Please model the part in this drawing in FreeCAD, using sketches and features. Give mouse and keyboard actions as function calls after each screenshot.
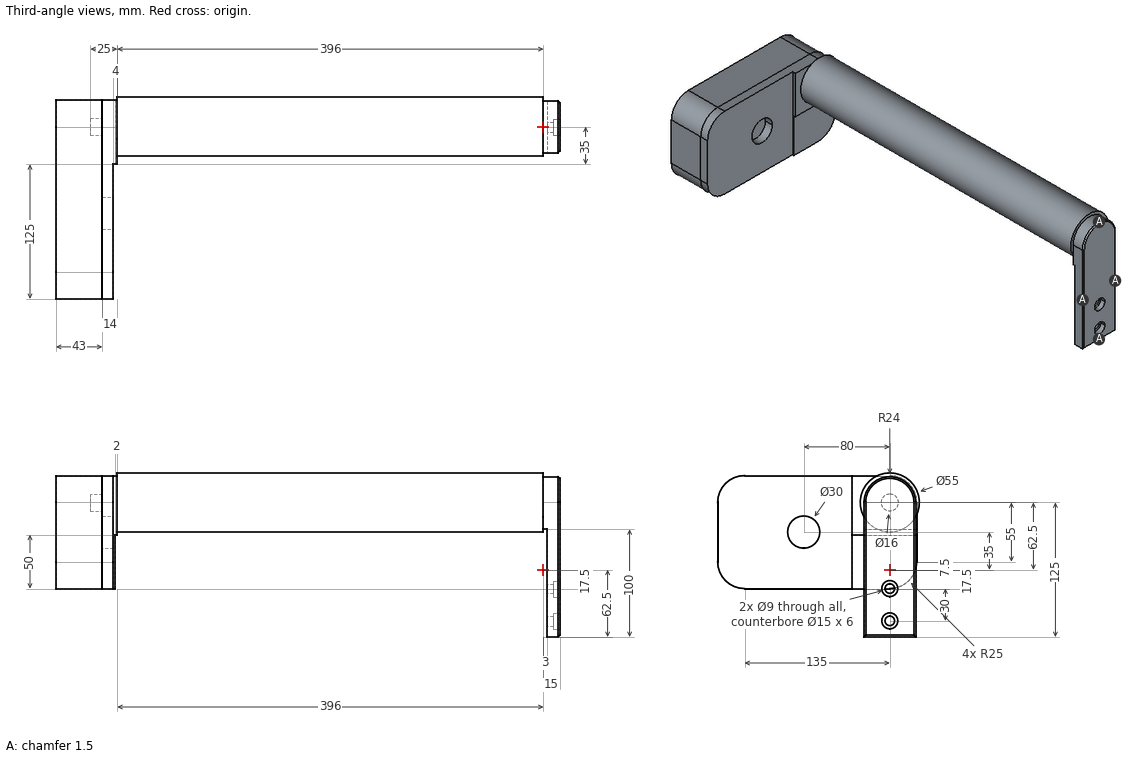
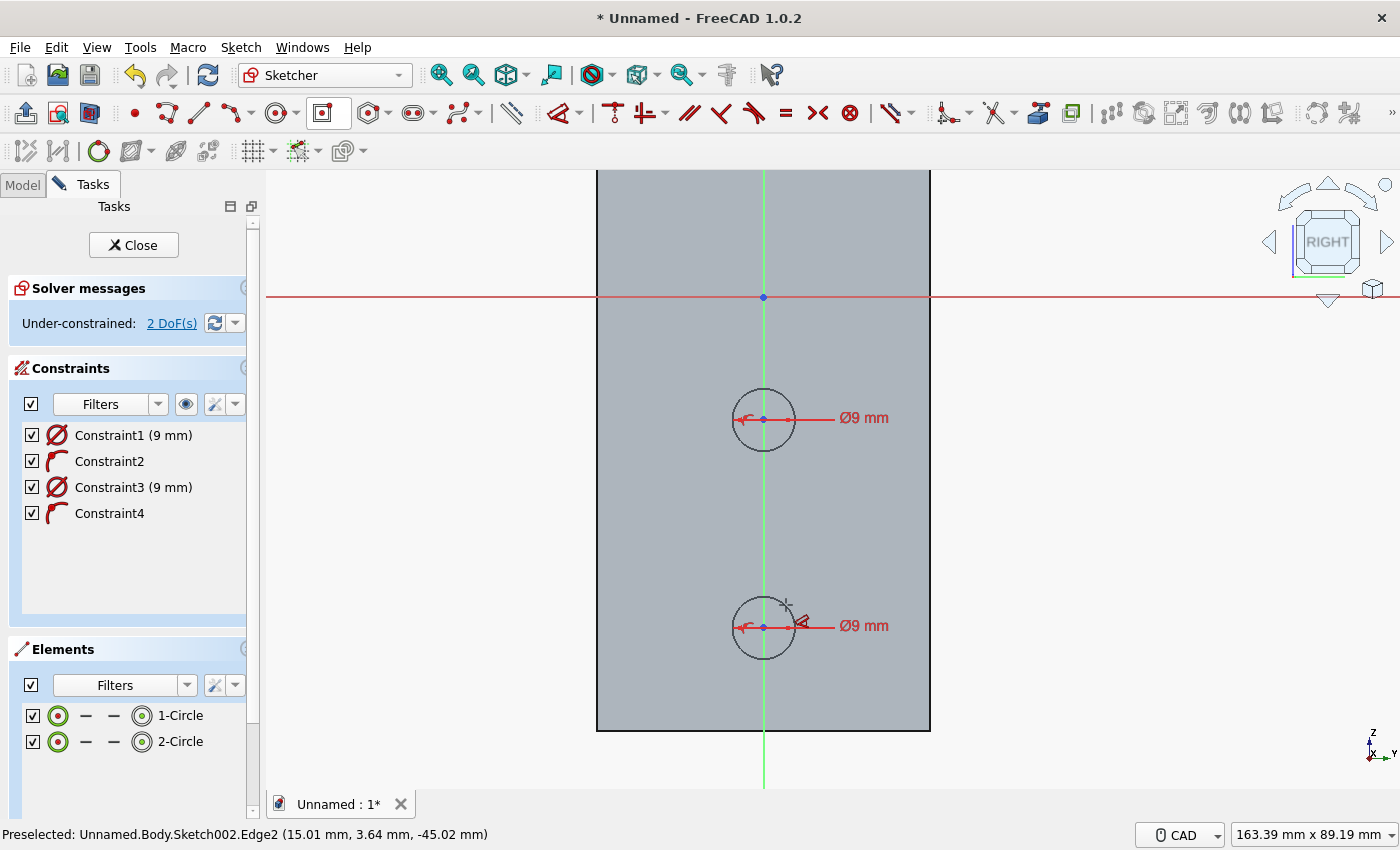
click(764, 420)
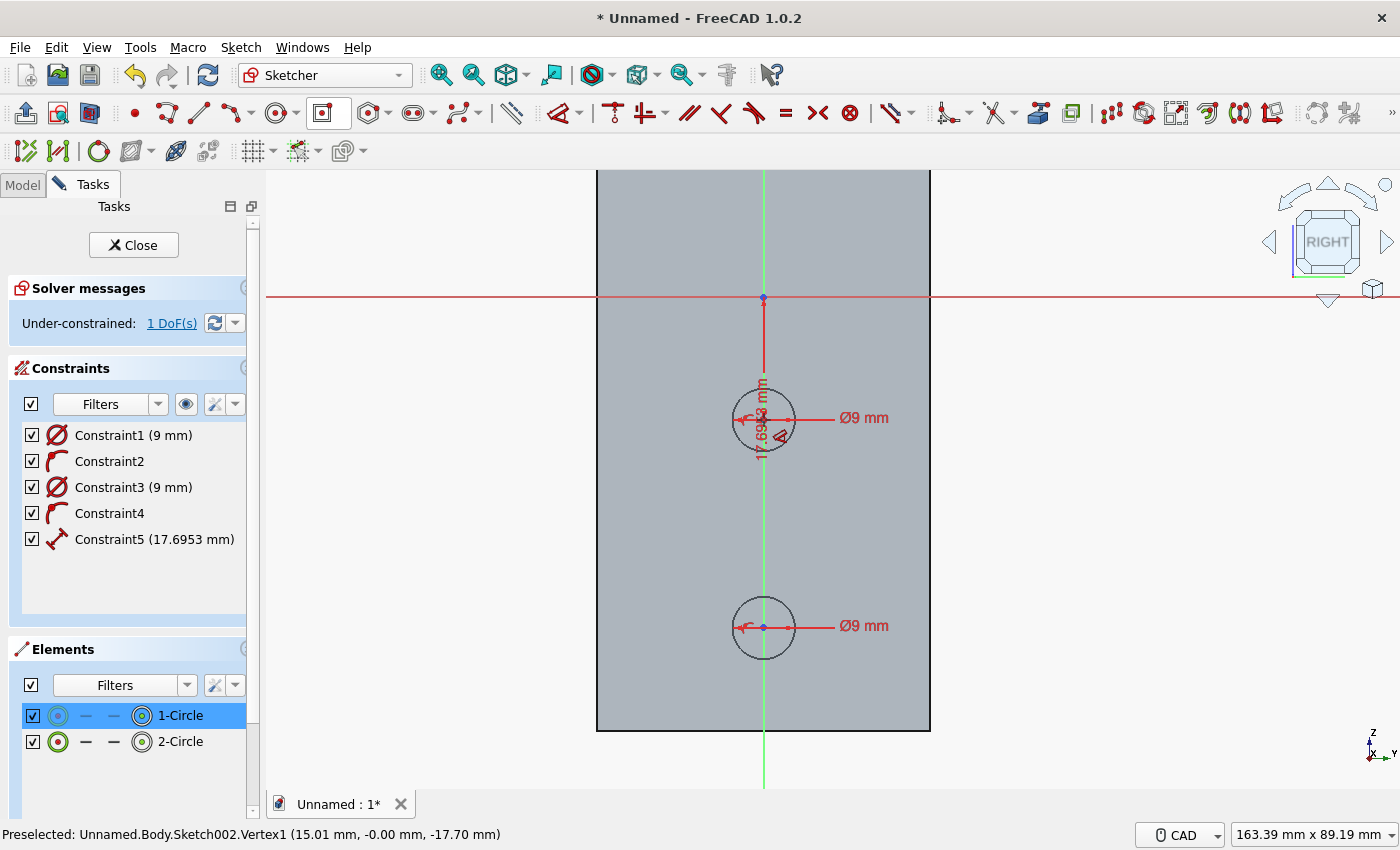
click(764, 628)
click(798, 524)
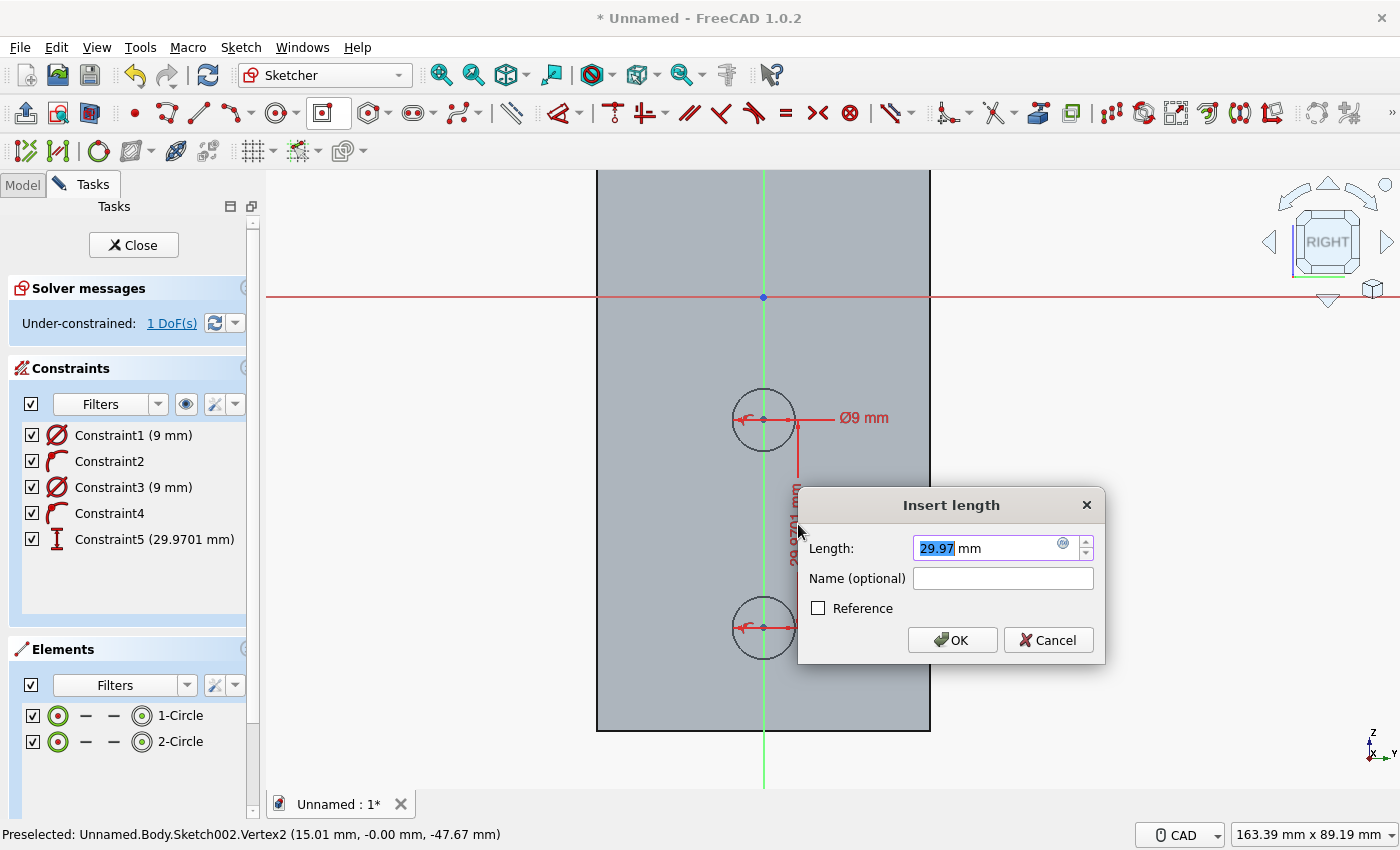
text(30)
key(Return)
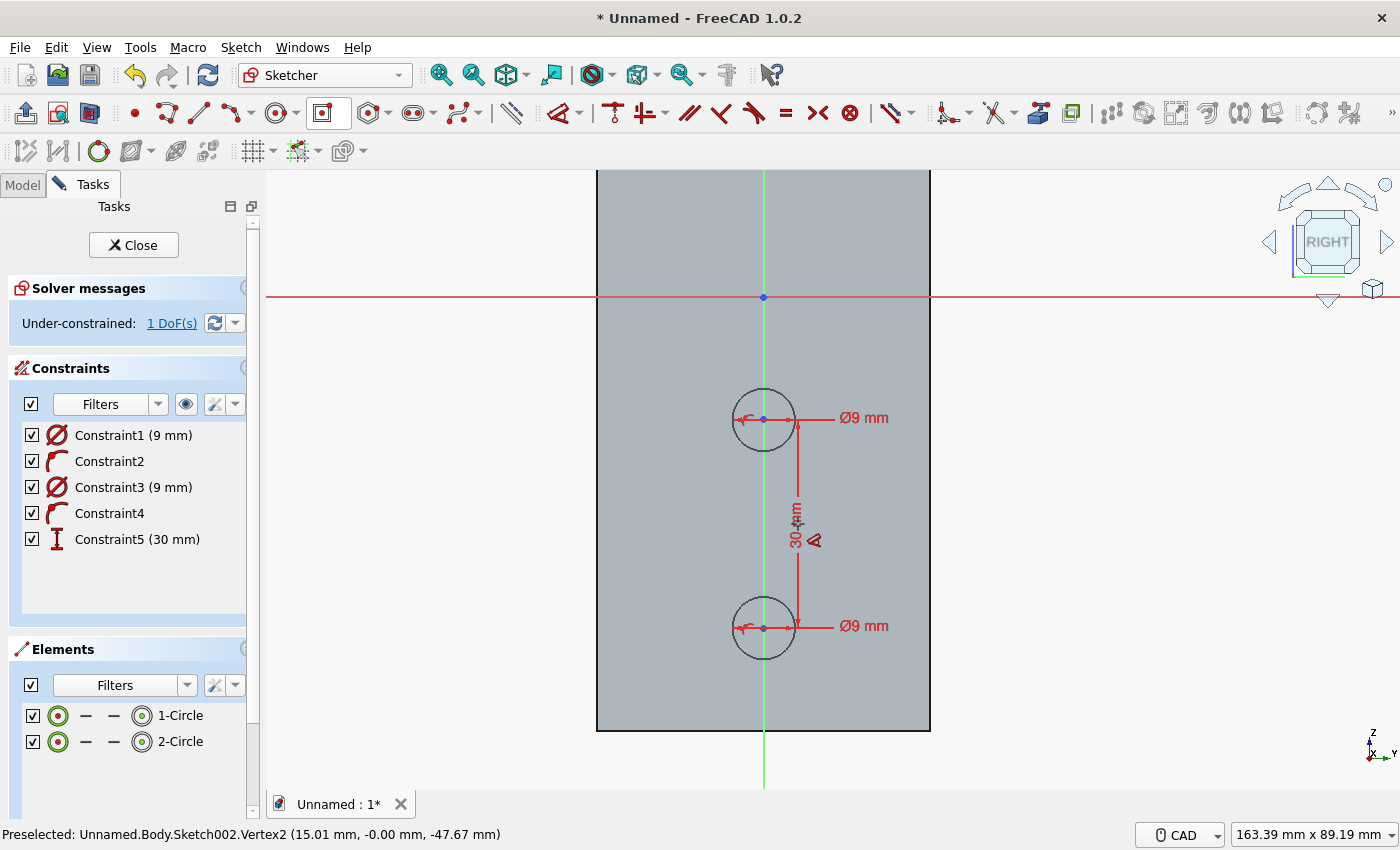
click(764, 420)
click(798, 359)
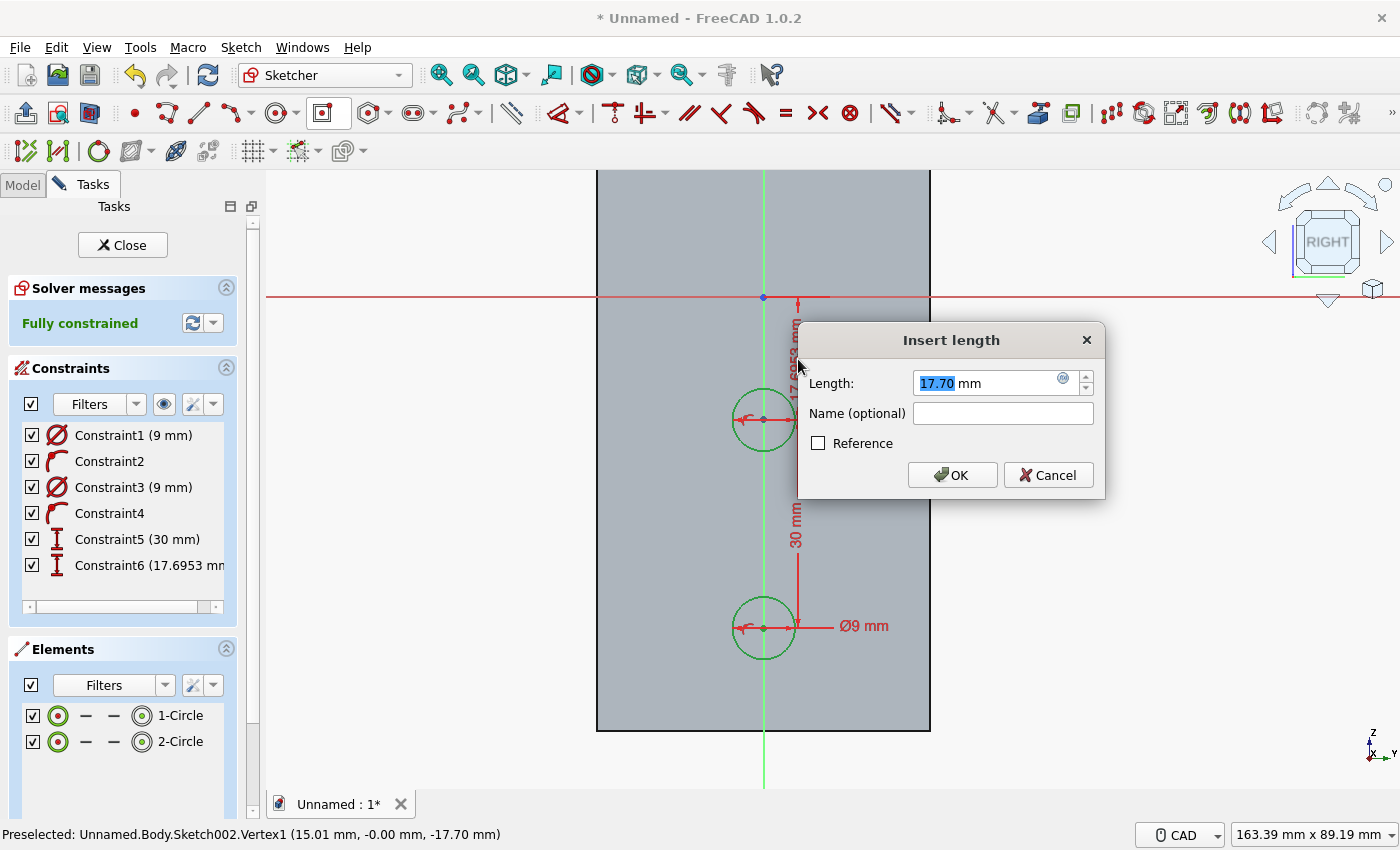
text(17.5)
key(Return)
key(Escape)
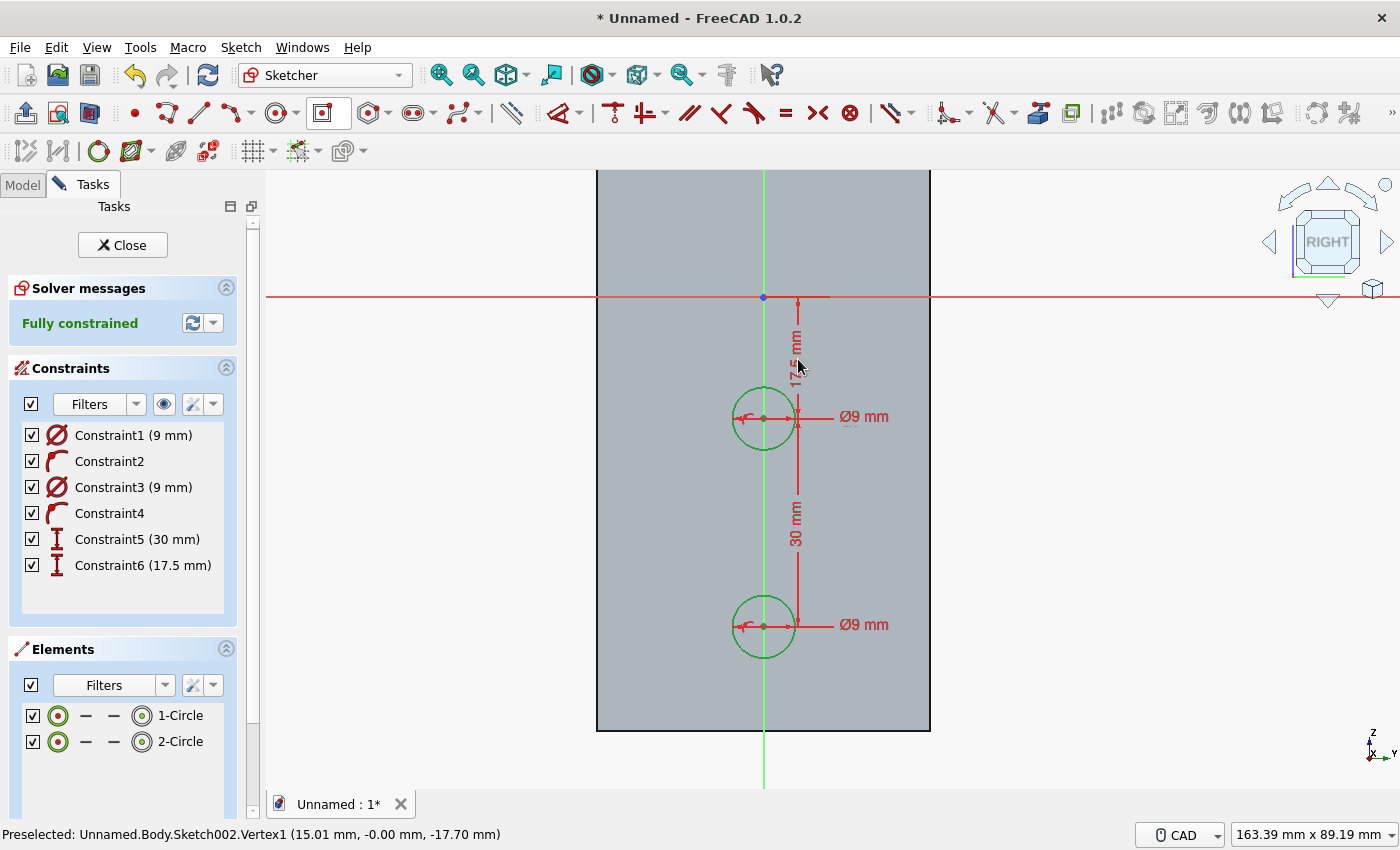
click(123, 245)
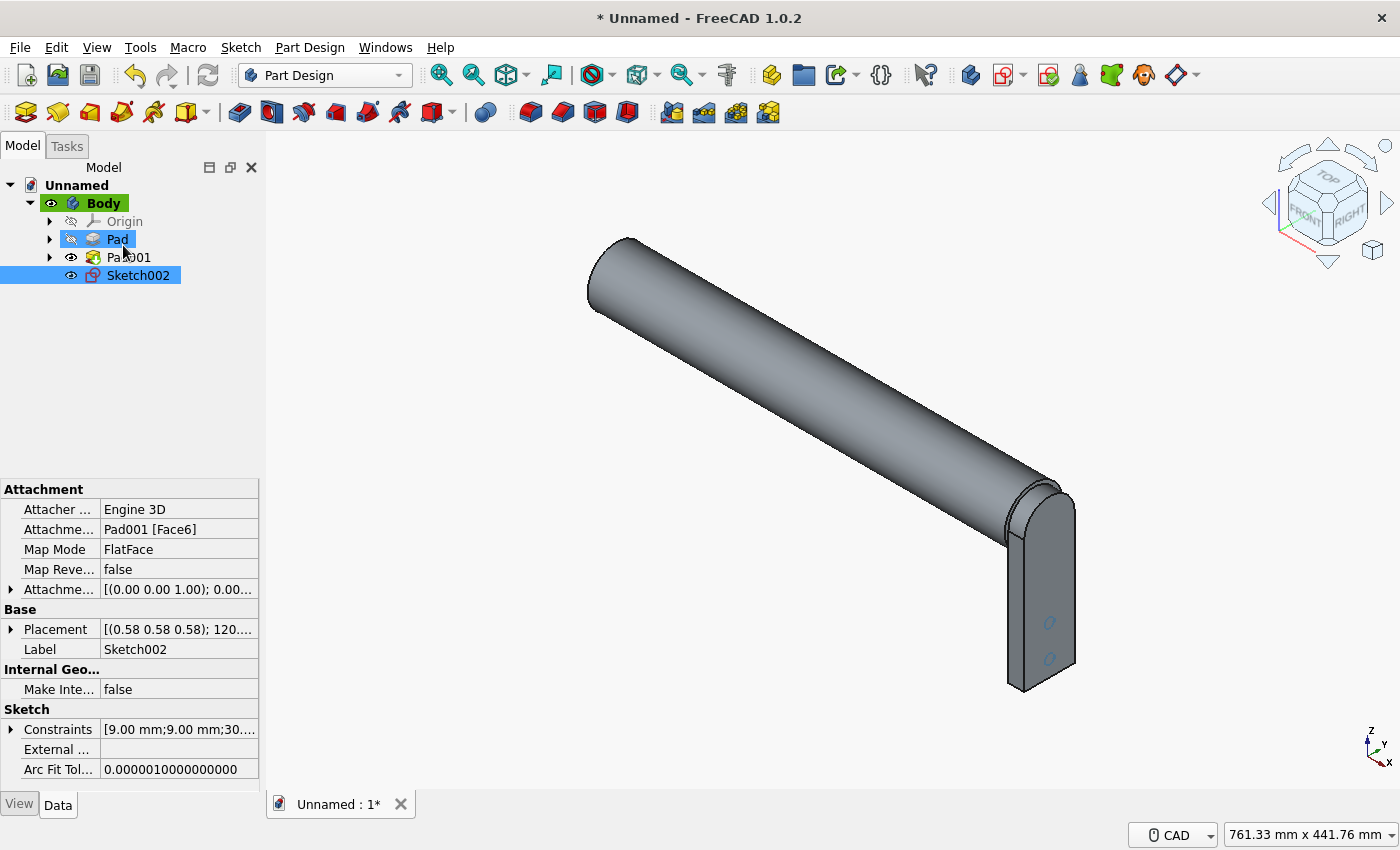
click(272, 112)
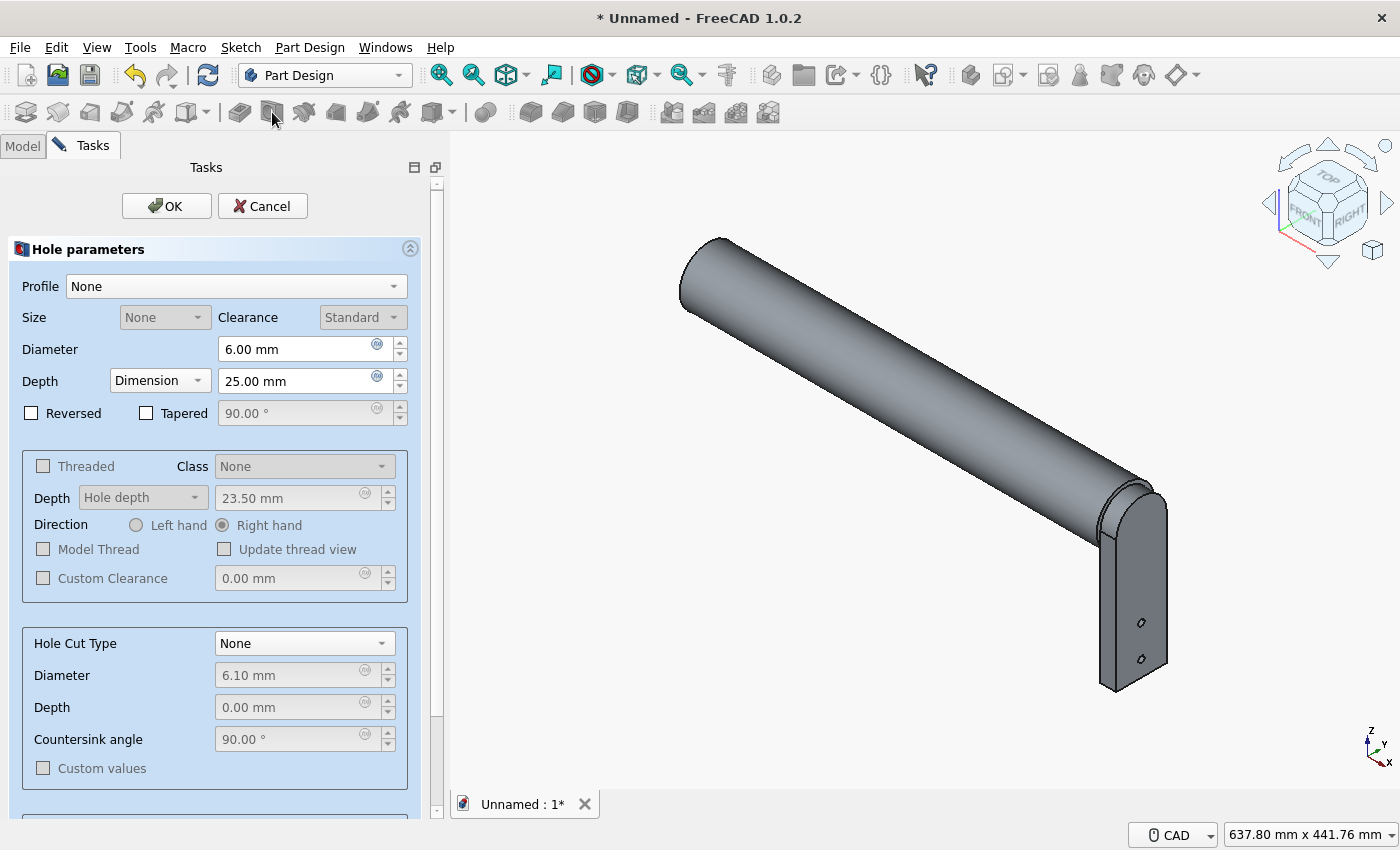
triple_click(305, 349)